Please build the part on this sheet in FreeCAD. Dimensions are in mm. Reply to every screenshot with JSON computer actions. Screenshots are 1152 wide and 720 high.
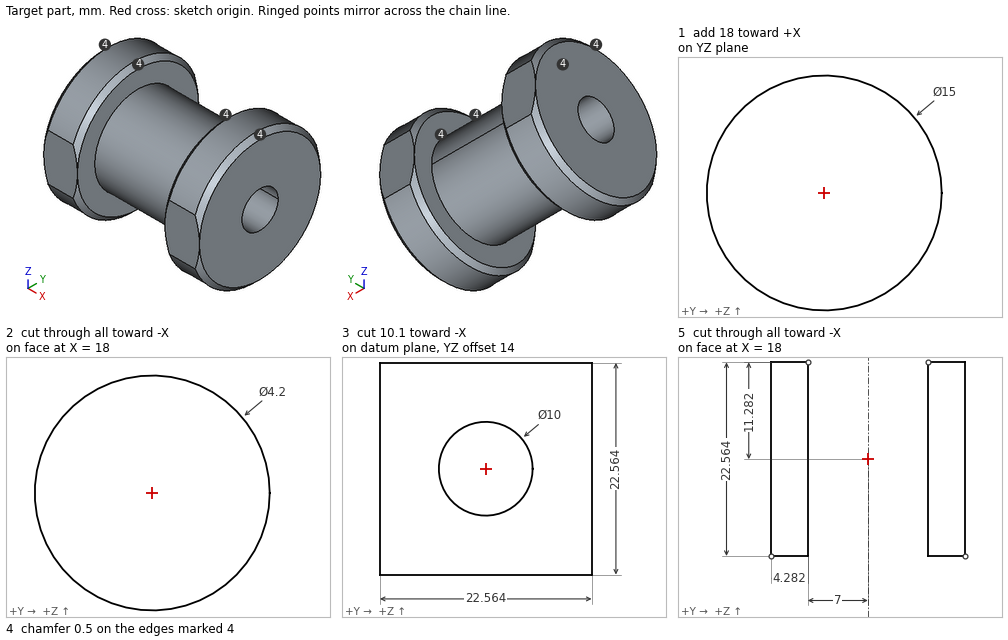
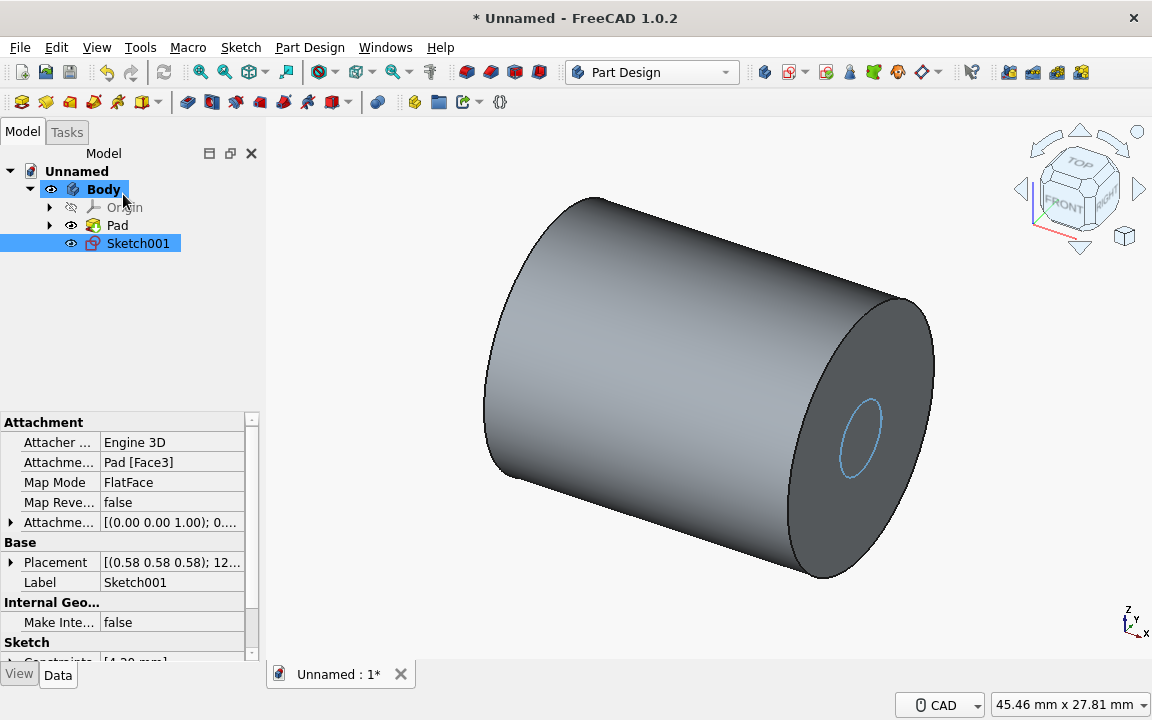
{"action": "left_click", "coordinate": [188, 102]}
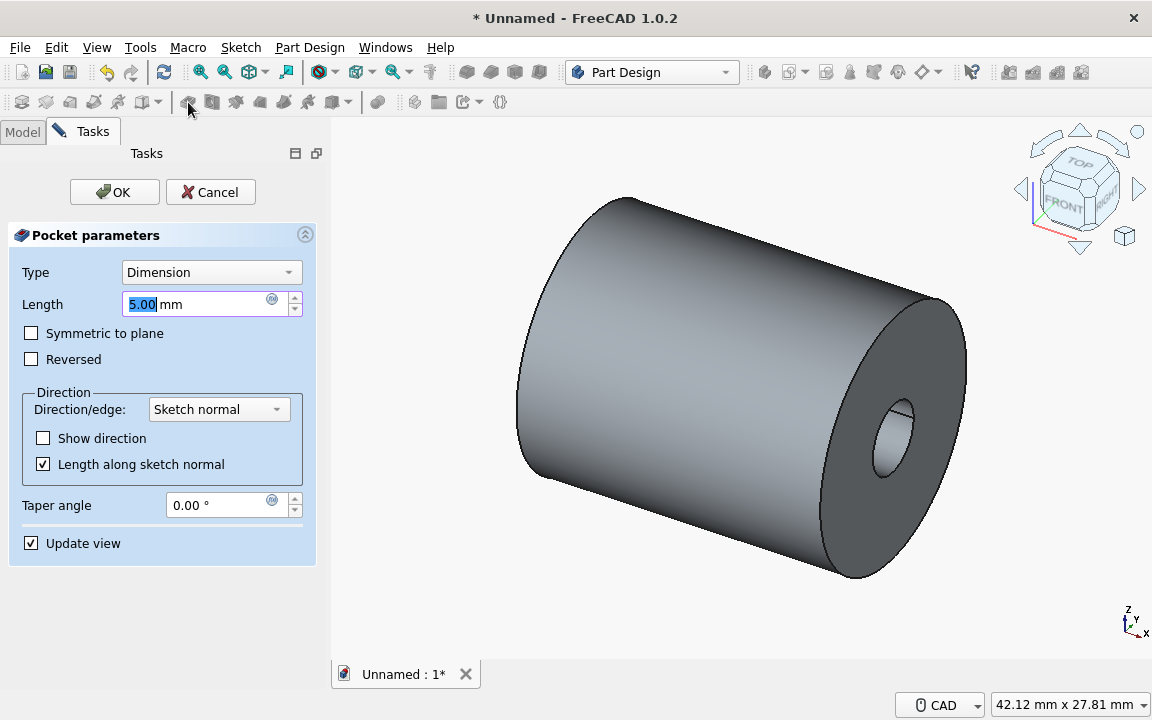
{"action": "left_click", "coordinate": [212, 272]}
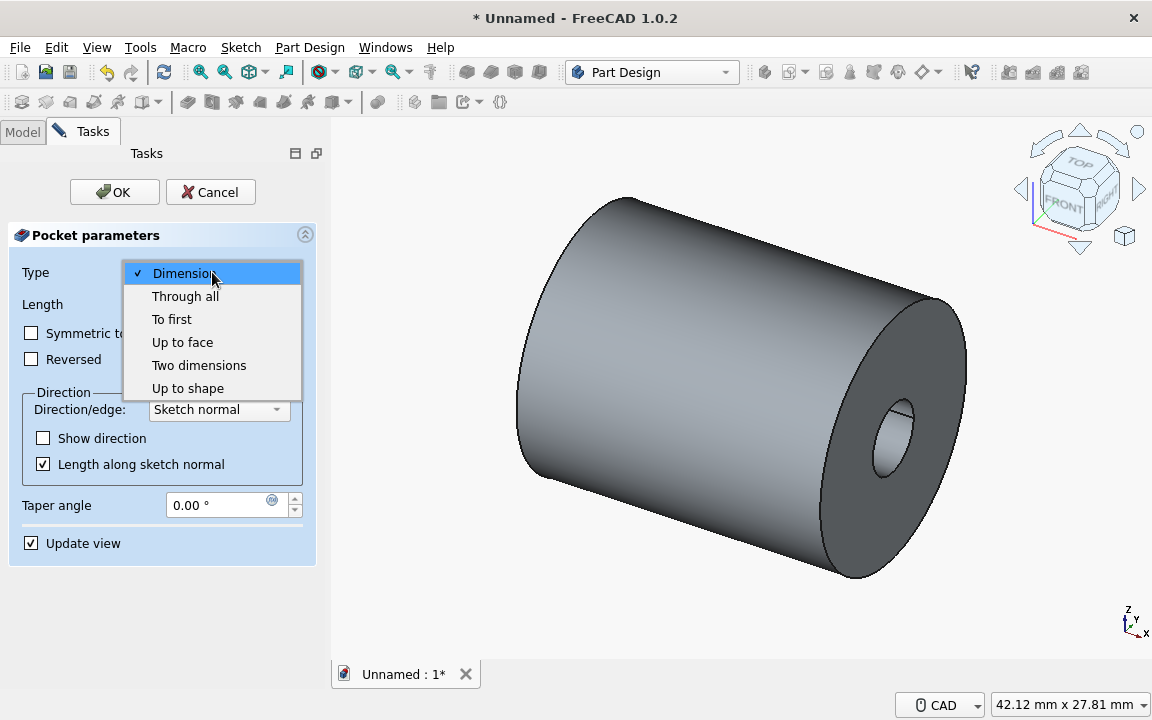
{"action": "left_click", "coordinate": [212, 296]}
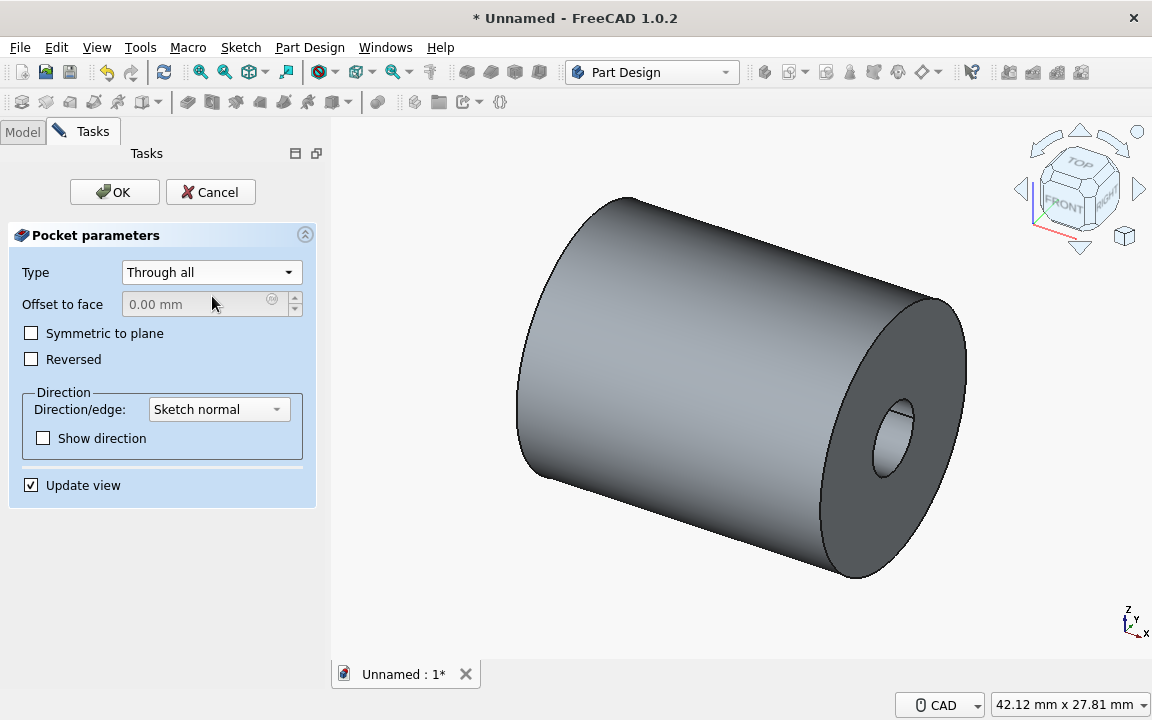
{"action": "left_click", "coordinate": [115, 192]}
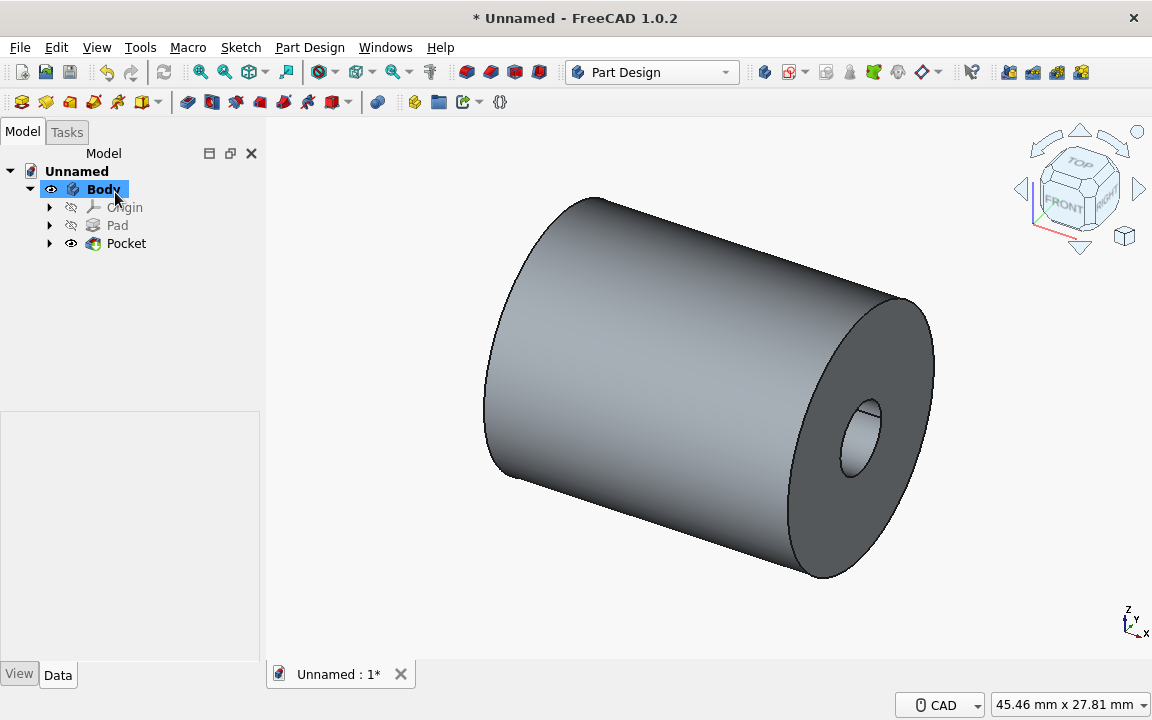
{"action": "left_click", "coordinate": [50, 207]}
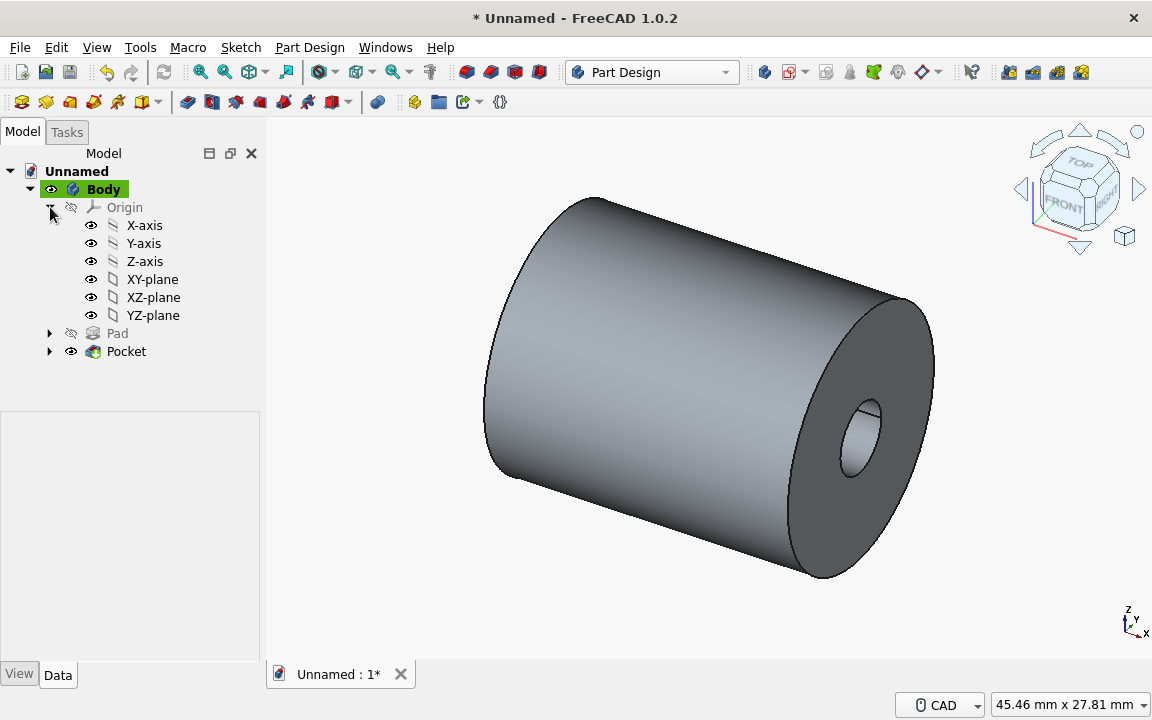
{"action": "left_click", "coordinate": [136, 315]}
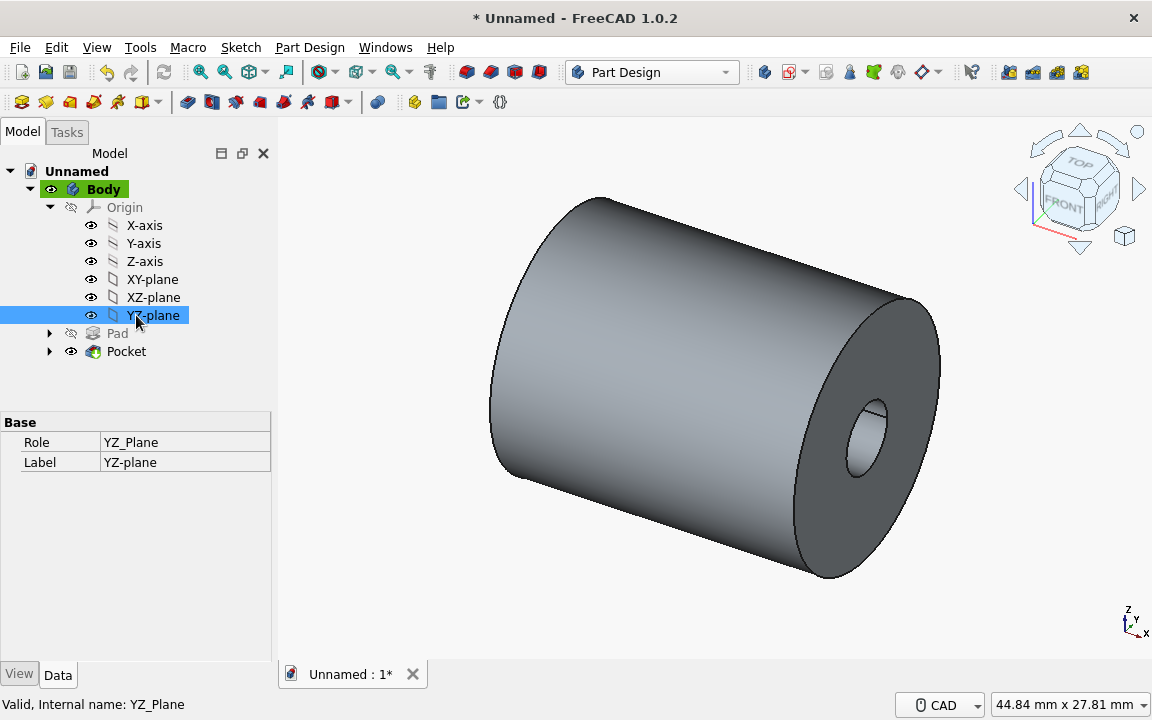
{"action": "left_click", "coordinate": [922, 72]}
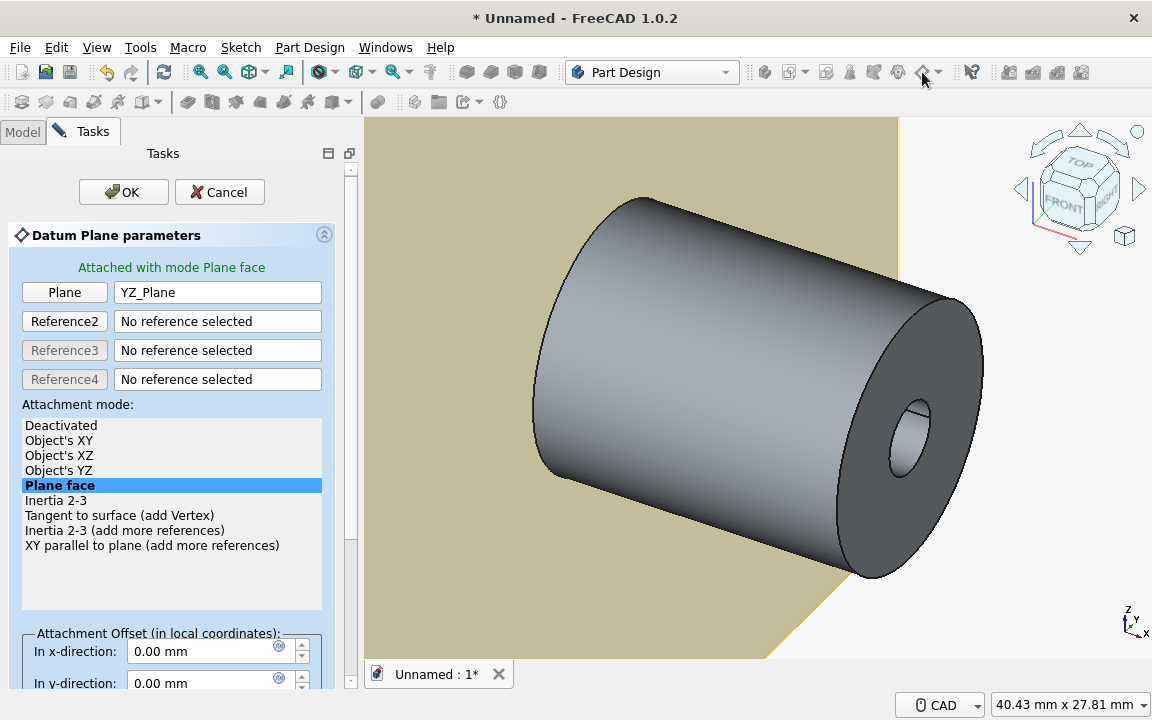
{"action": "scroll", "coordinate": [351, 426], "scroll_direction": "down", "scroll_amount": 2}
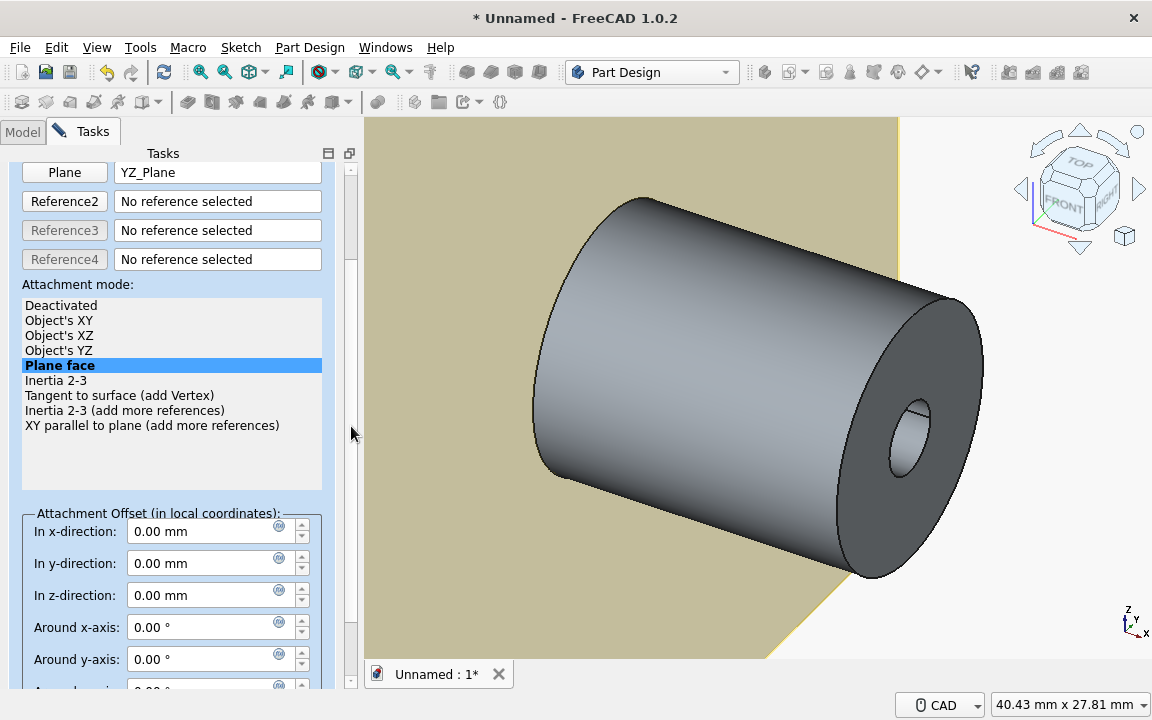
{"action": "triple_click", "coordinate": [210, 595]}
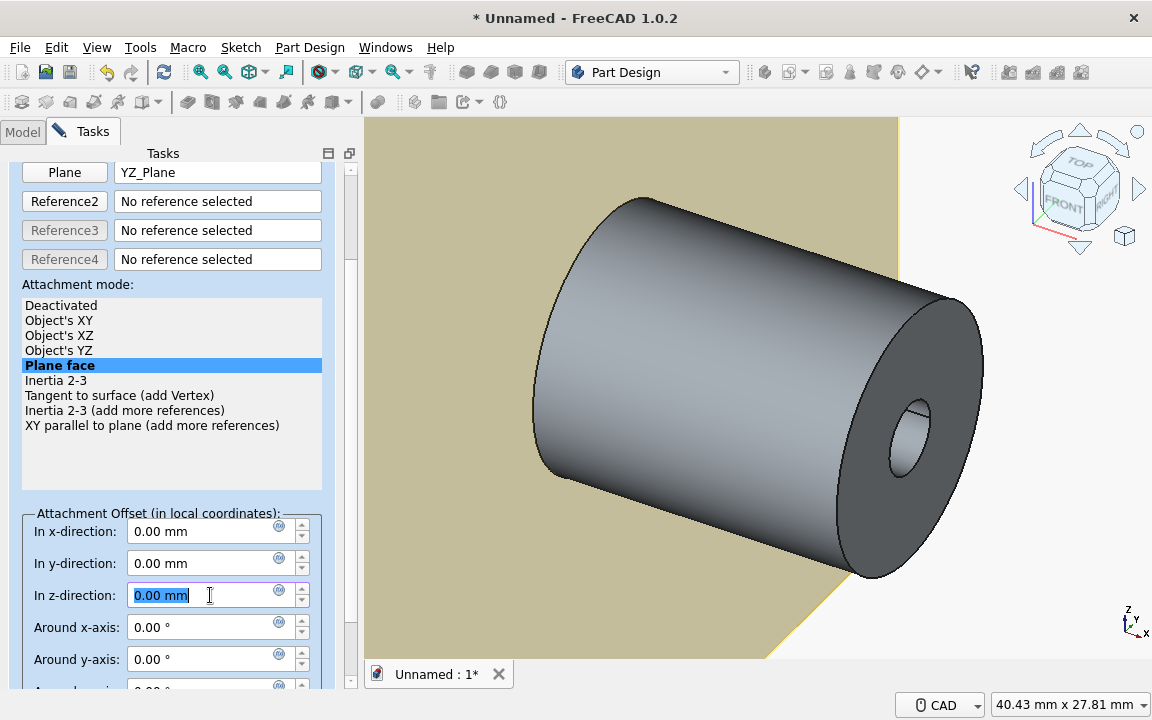
{"action": "type", "text": "14"}
{"action": "key", "text": "Tab"}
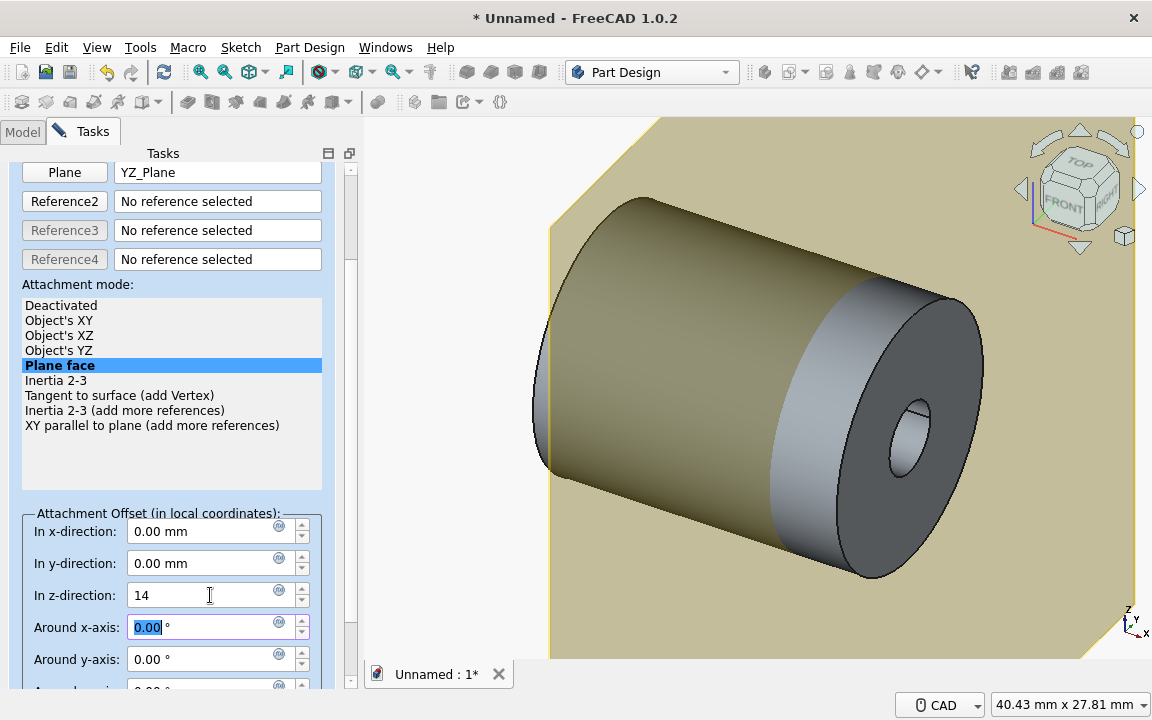
{"action": "scroll", "coordinate": [351, 426], "scroll_direction": "up", "scroll_amount": 3}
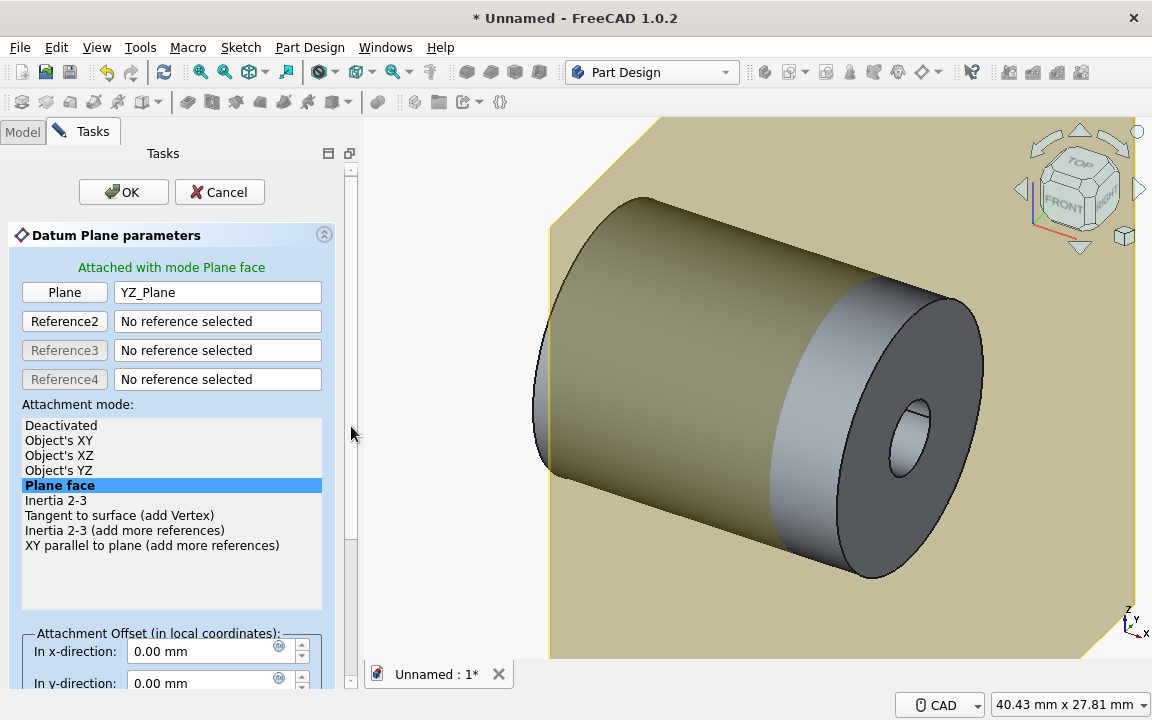
{"action": "left_click", "coordinate": [124, 192]}